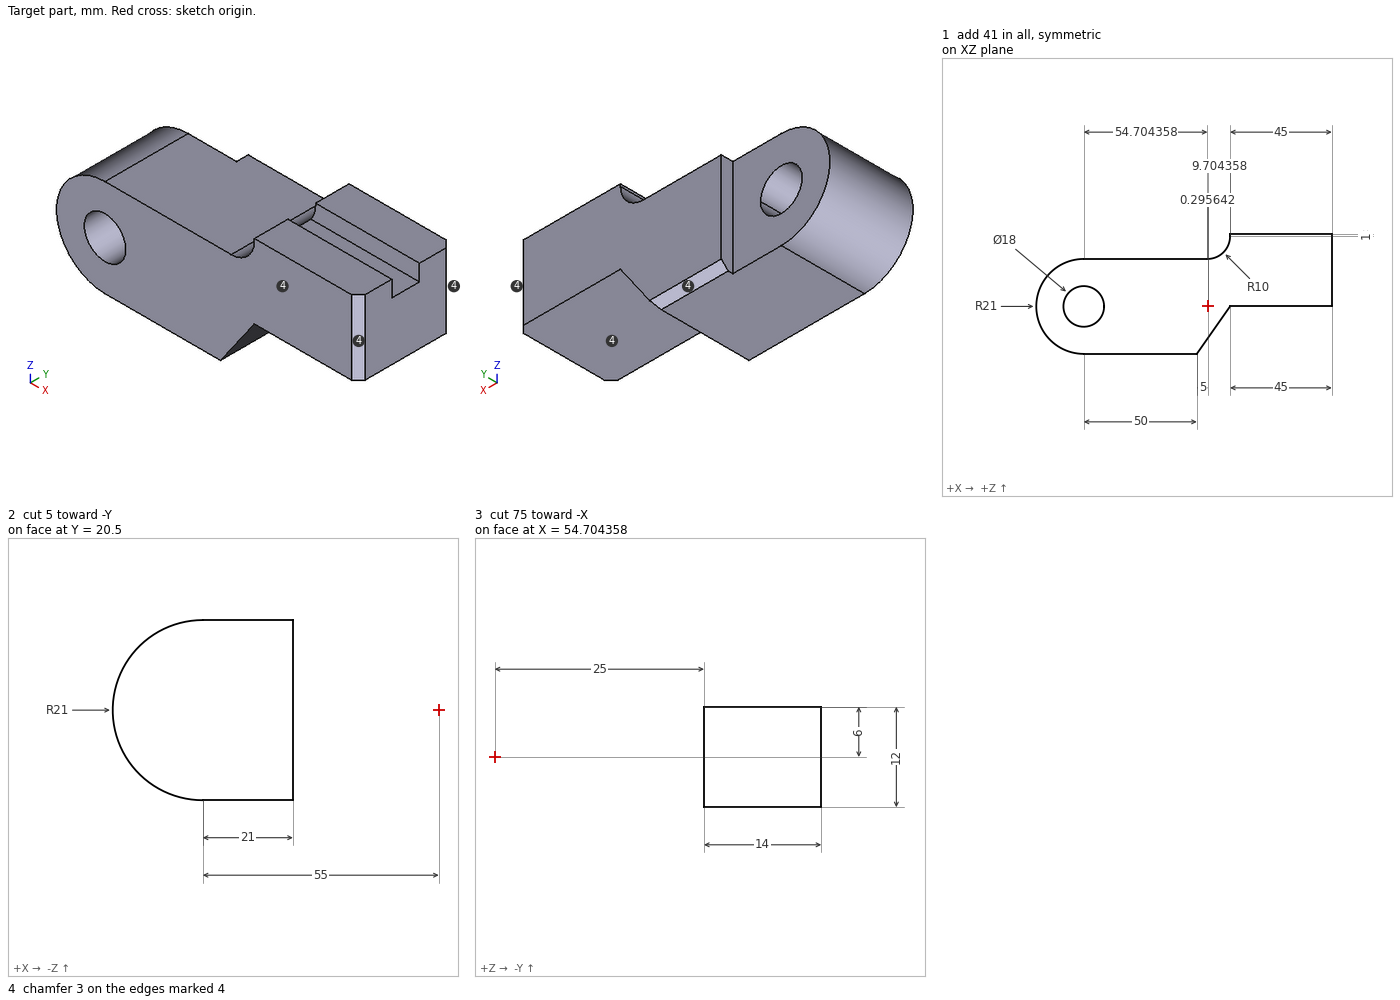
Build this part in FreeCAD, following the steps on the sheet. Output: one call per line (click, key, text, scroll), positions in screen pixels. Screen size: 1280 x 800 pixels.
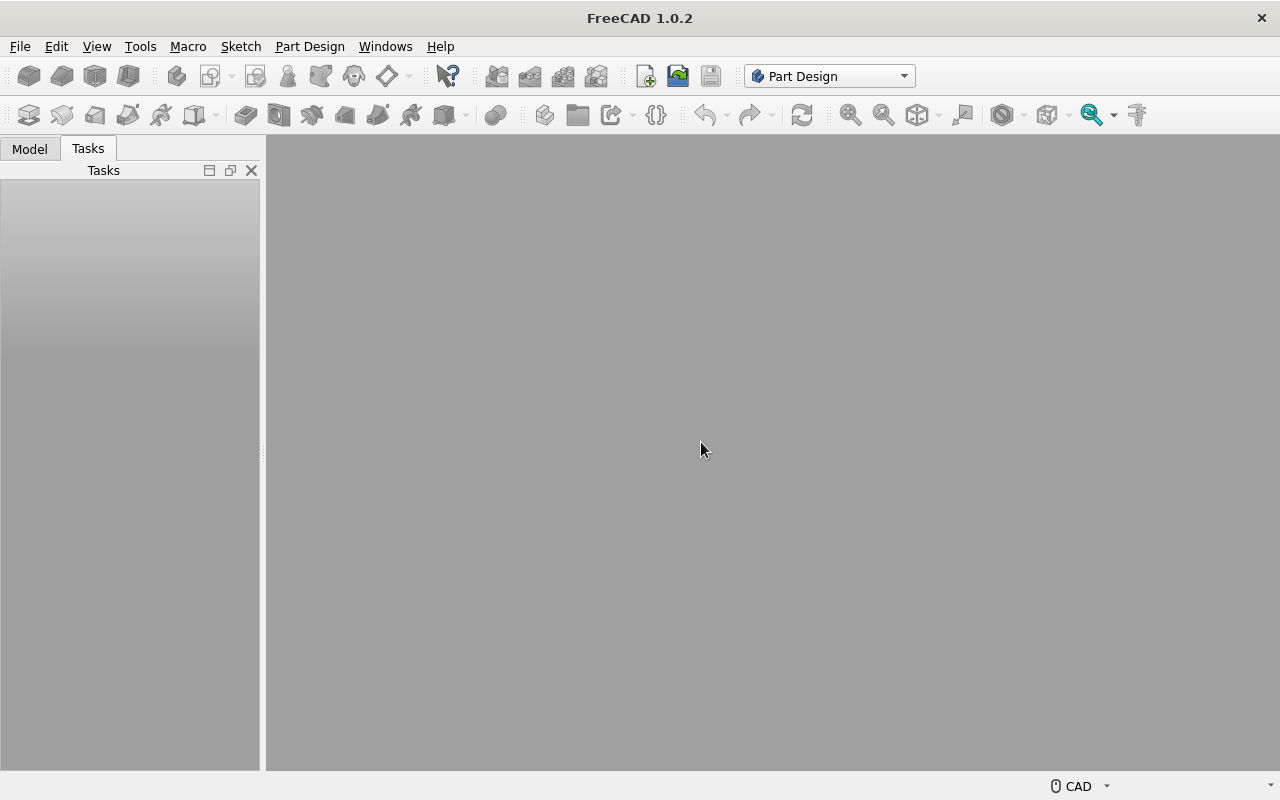
click(645, 76)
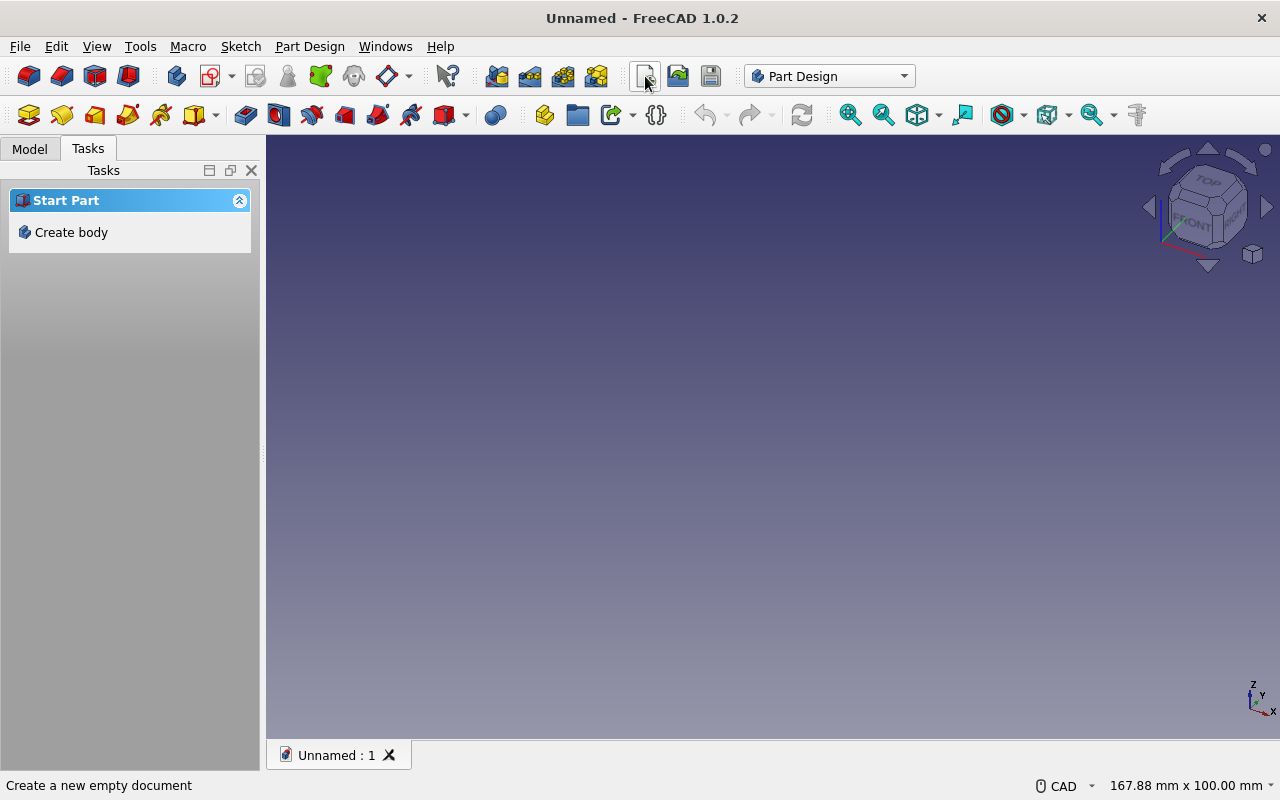
click(210, 76)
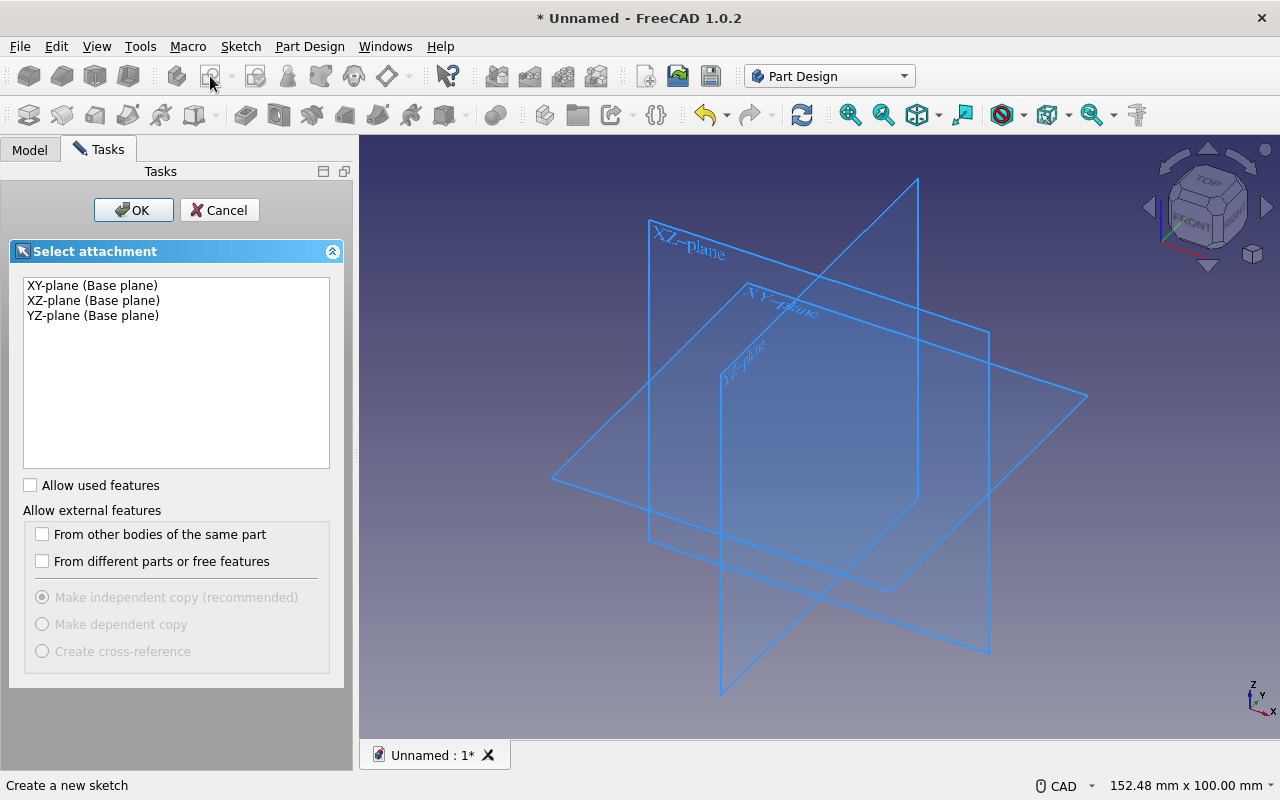
click(84, 300)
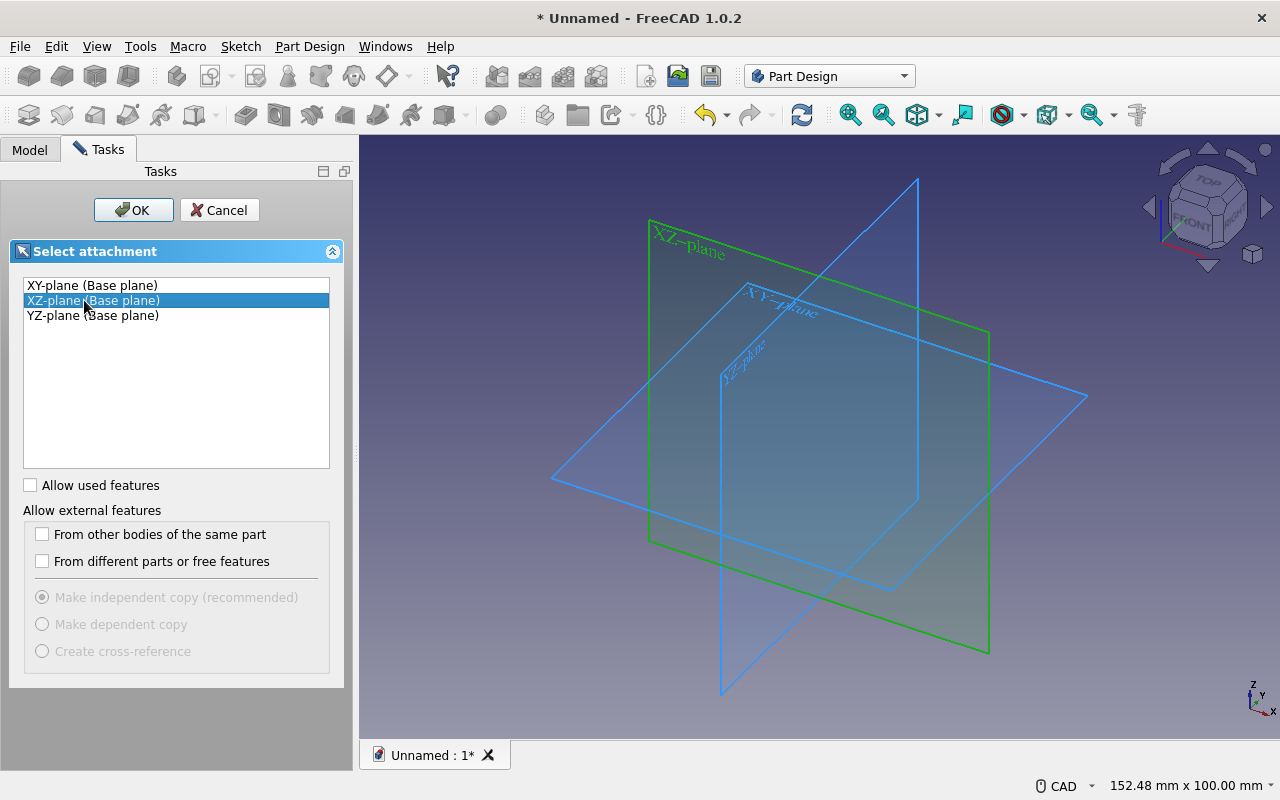
click(134, 210)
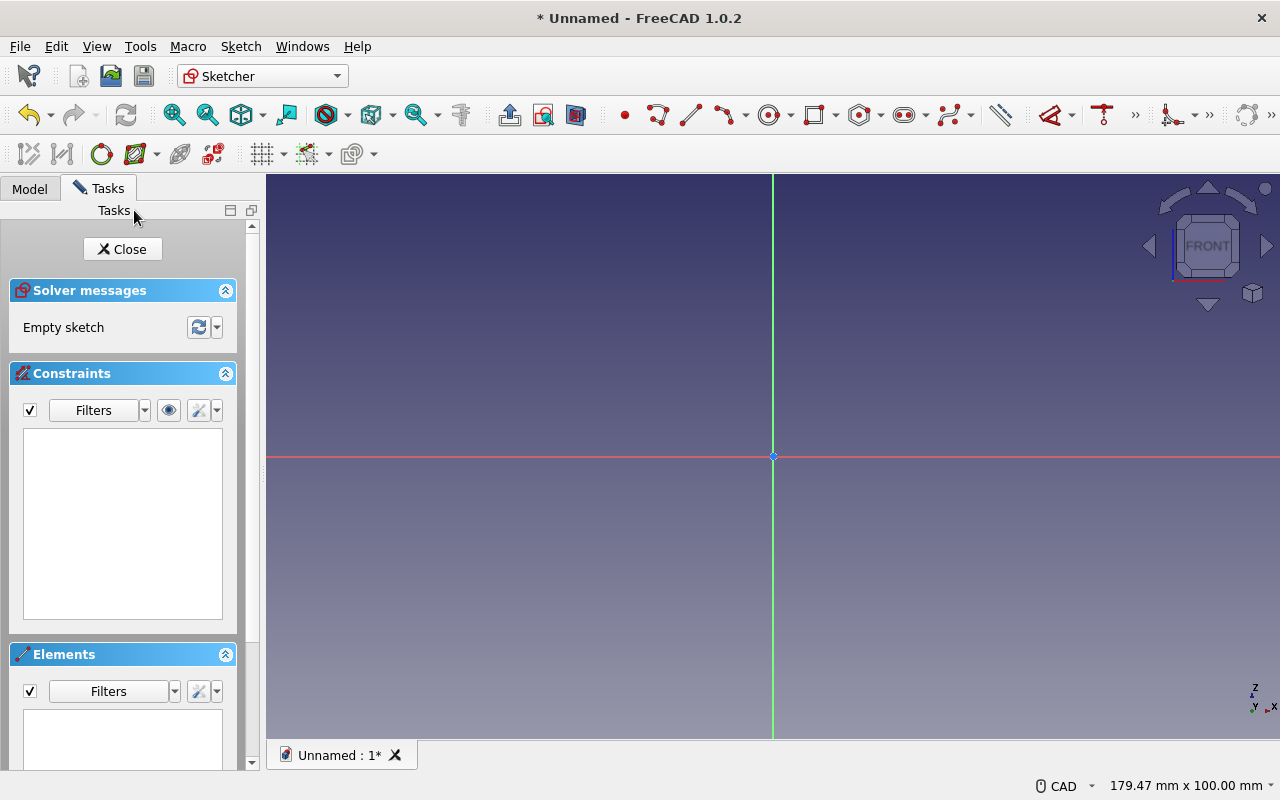
click(691, 116)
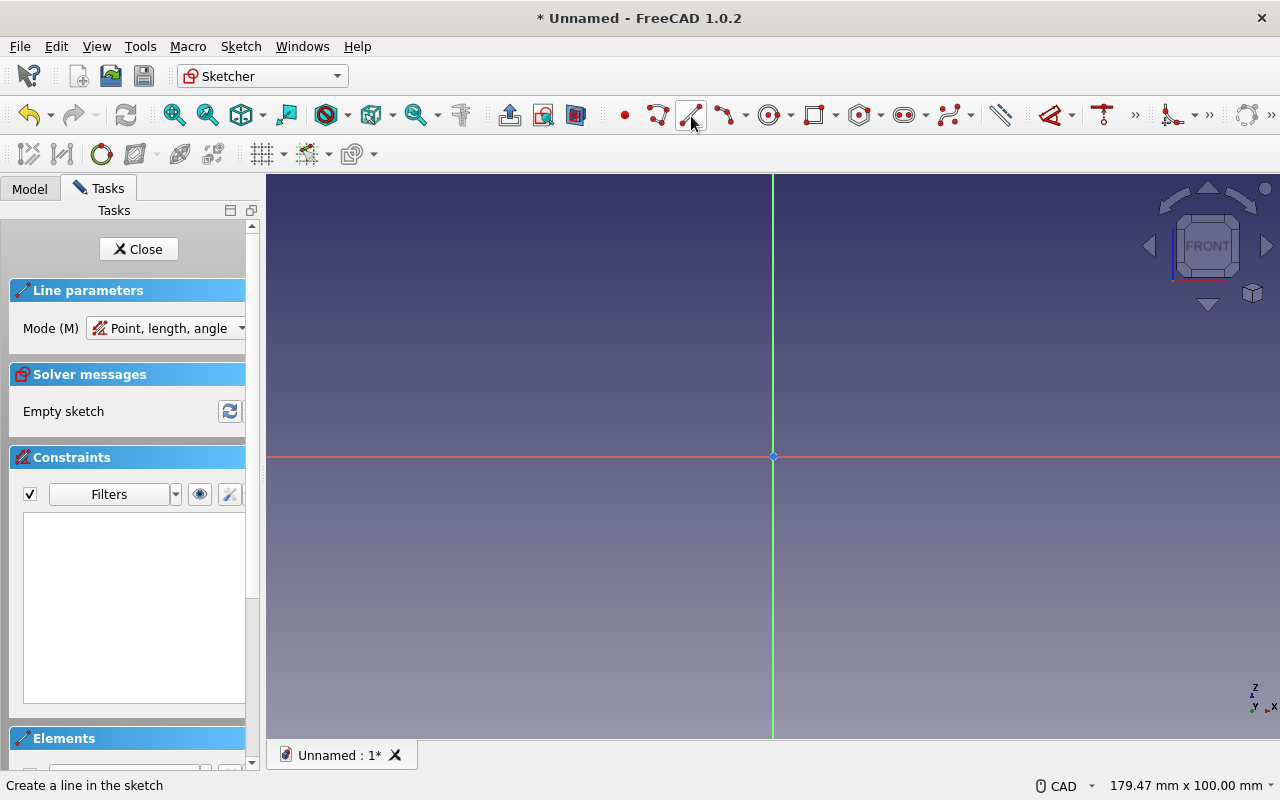
click(462, 338)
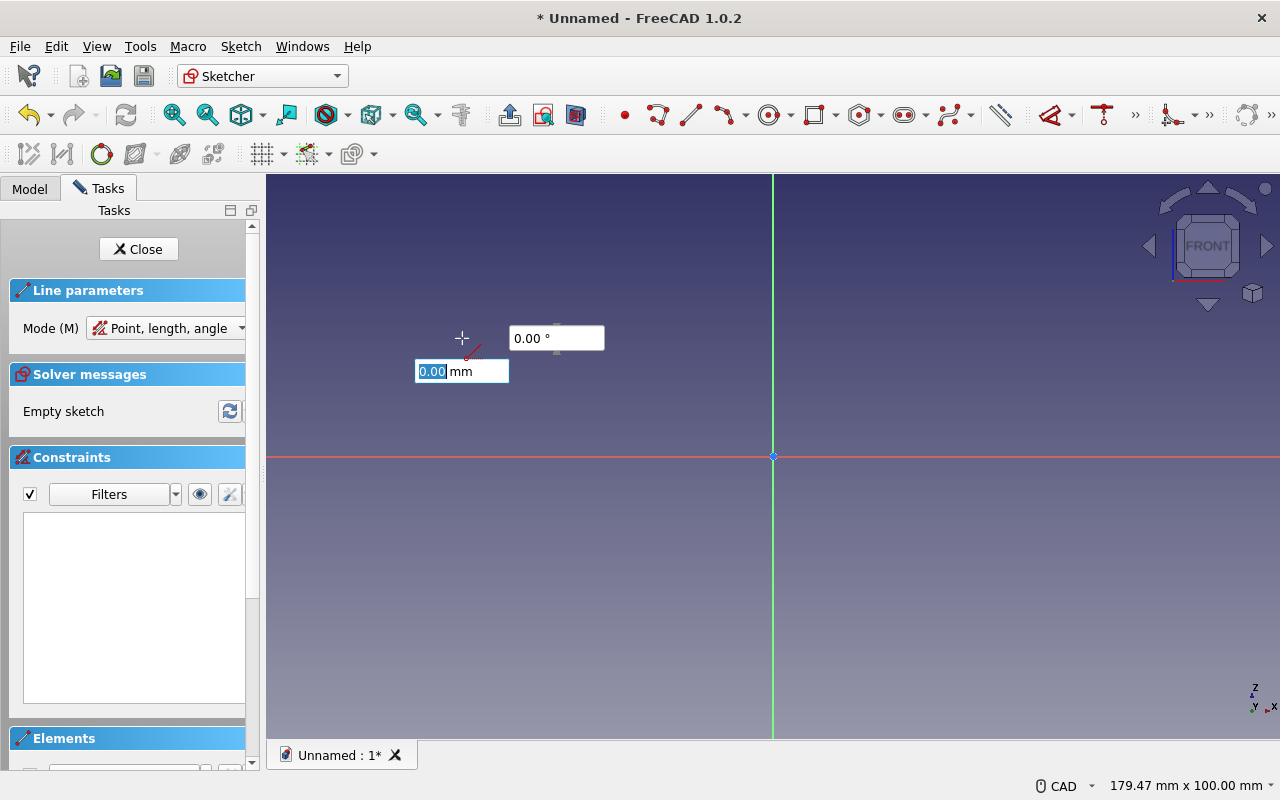
scroll(771, 338, up, 12)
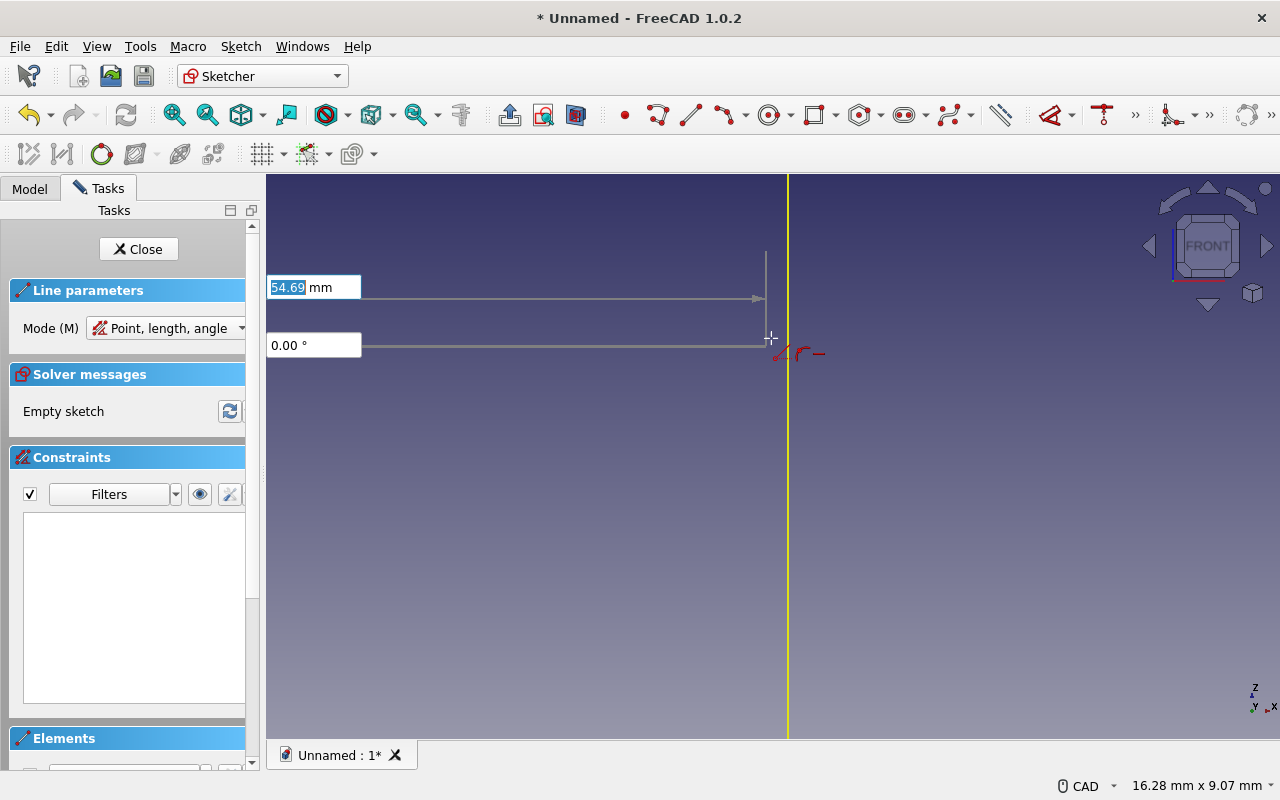
click(770, 335)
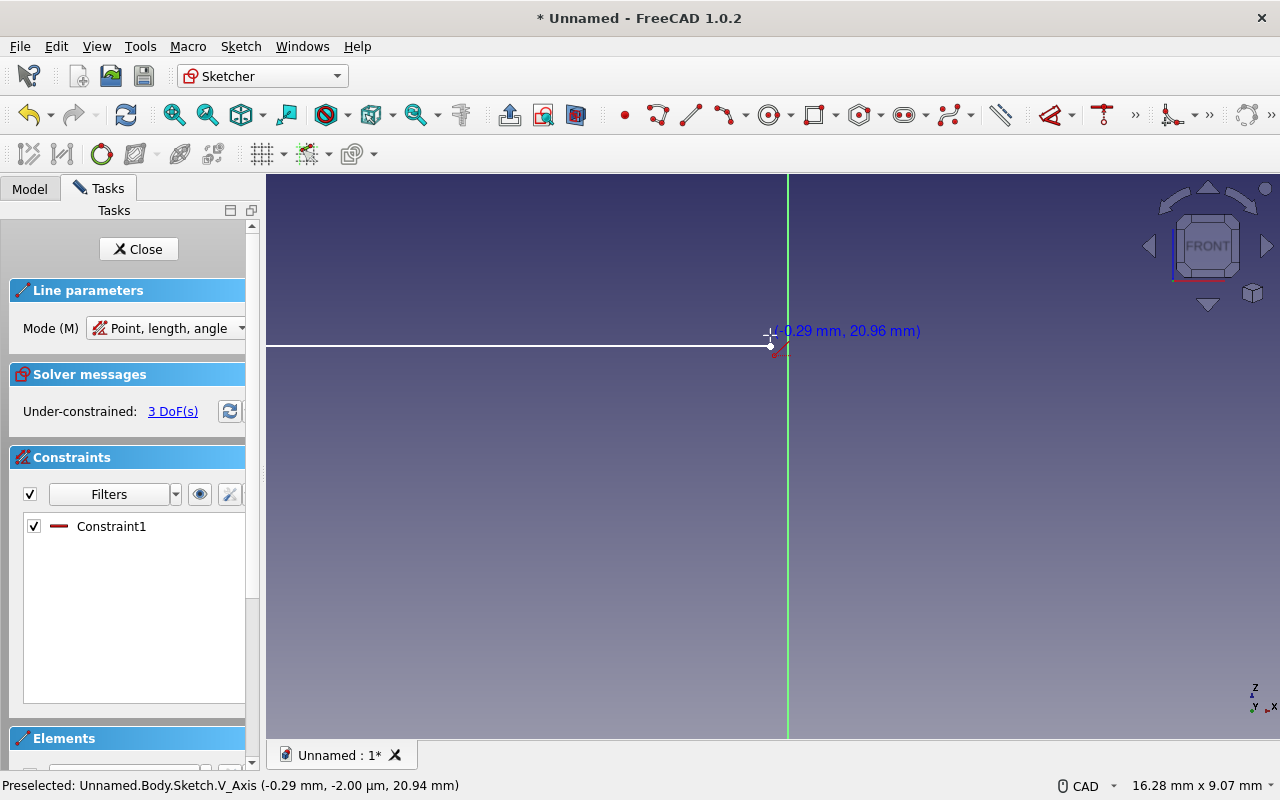
click(658, 116)